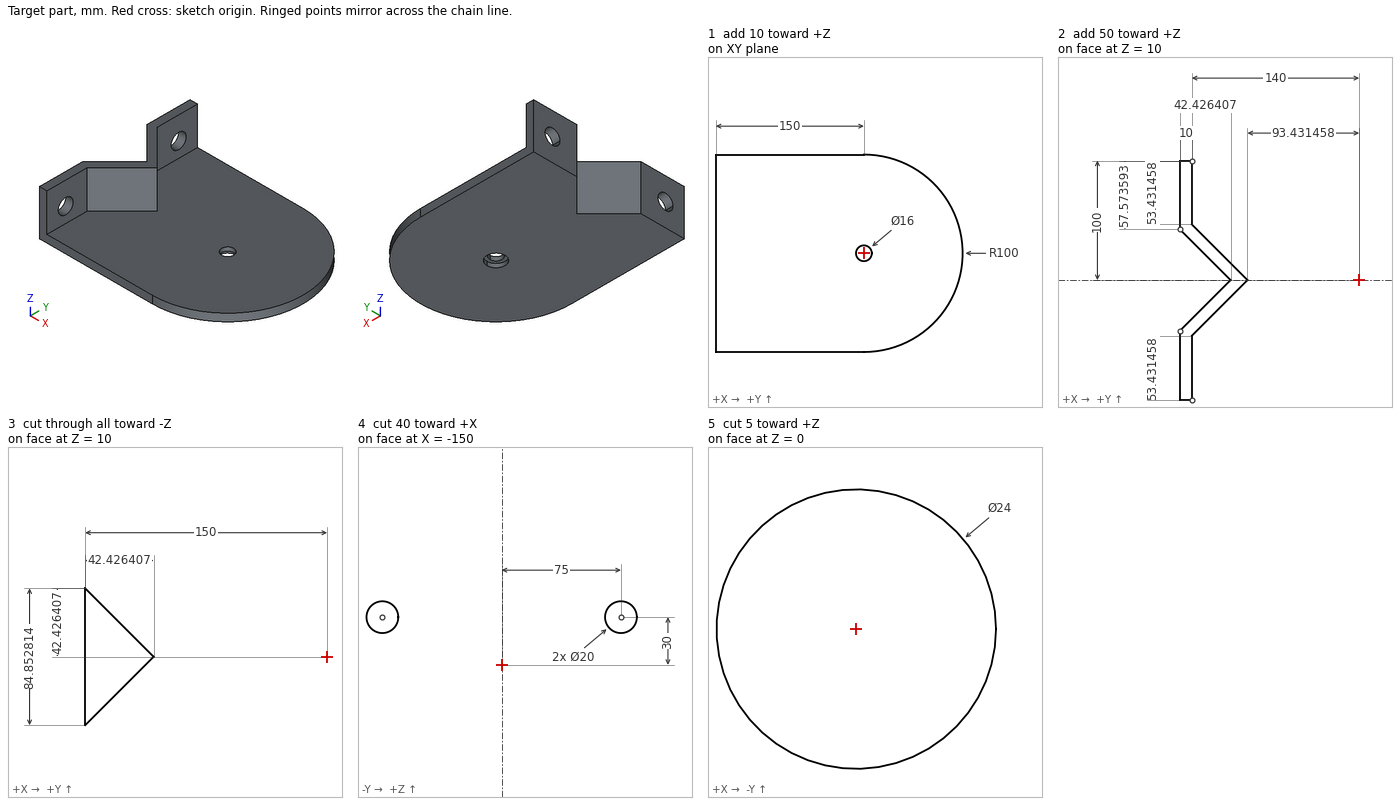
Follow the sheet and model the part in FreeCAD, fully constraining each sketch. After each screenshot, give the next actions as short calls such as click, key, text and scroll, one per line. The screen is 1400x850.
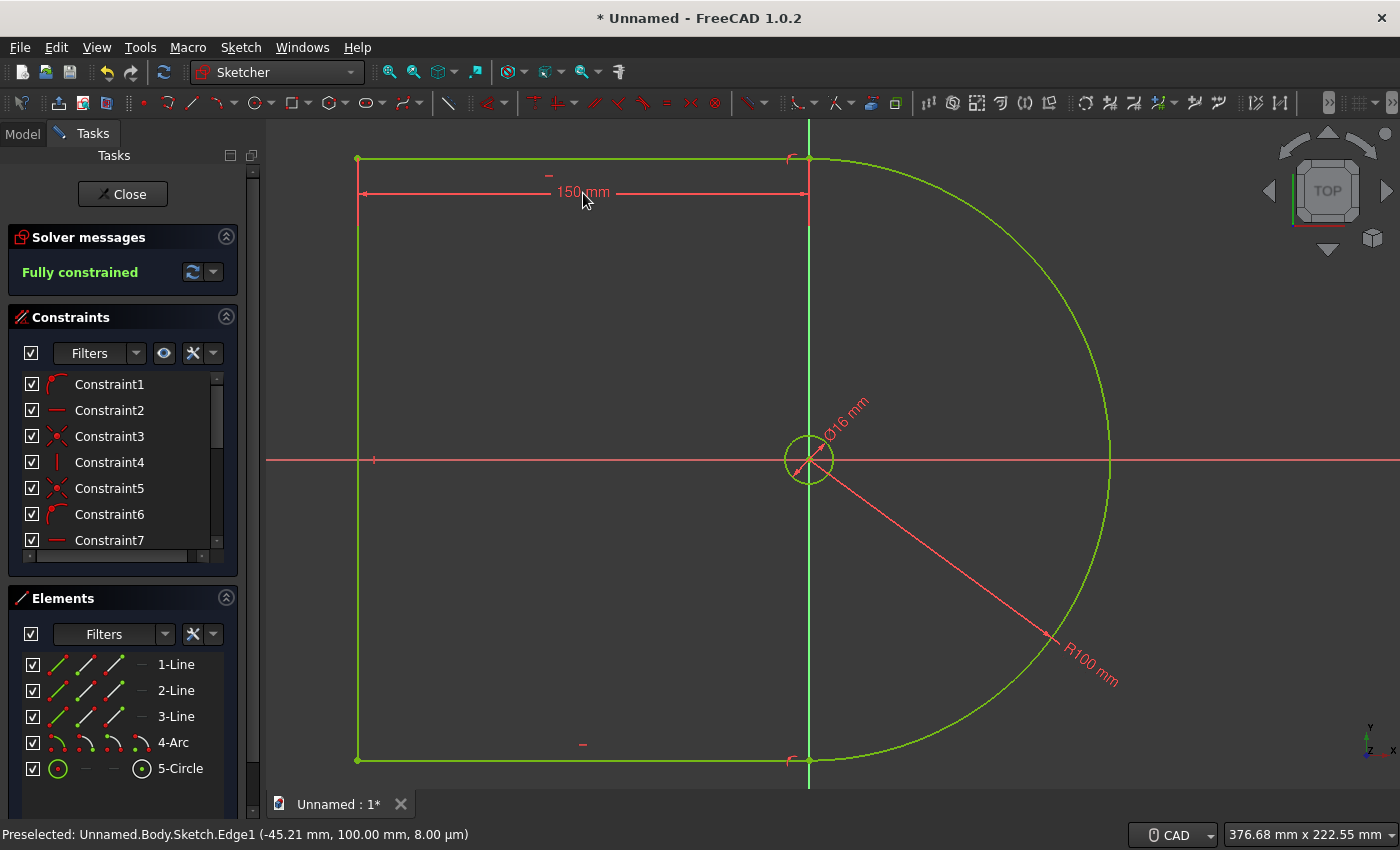
click(123, 194)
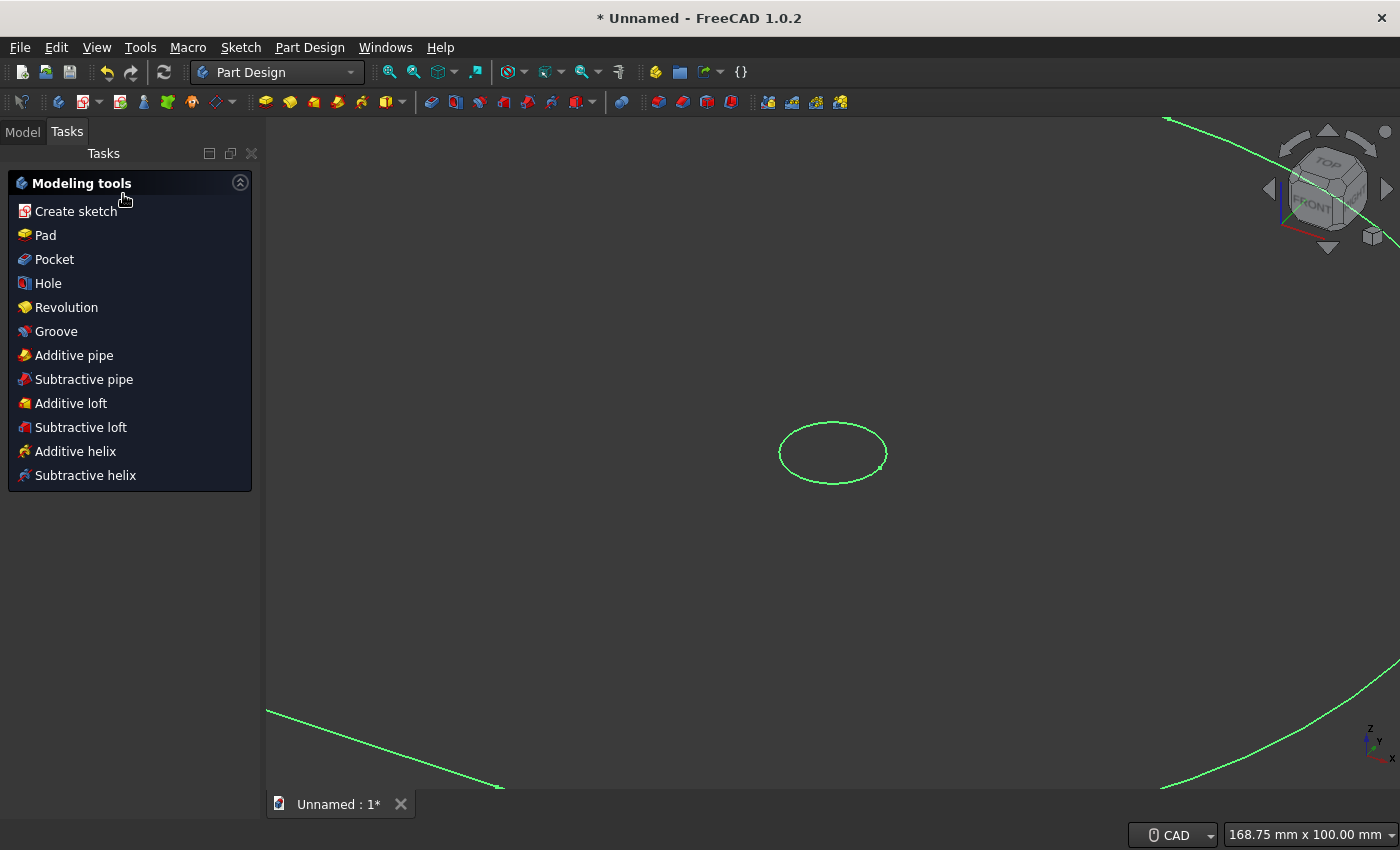
click(266, 102)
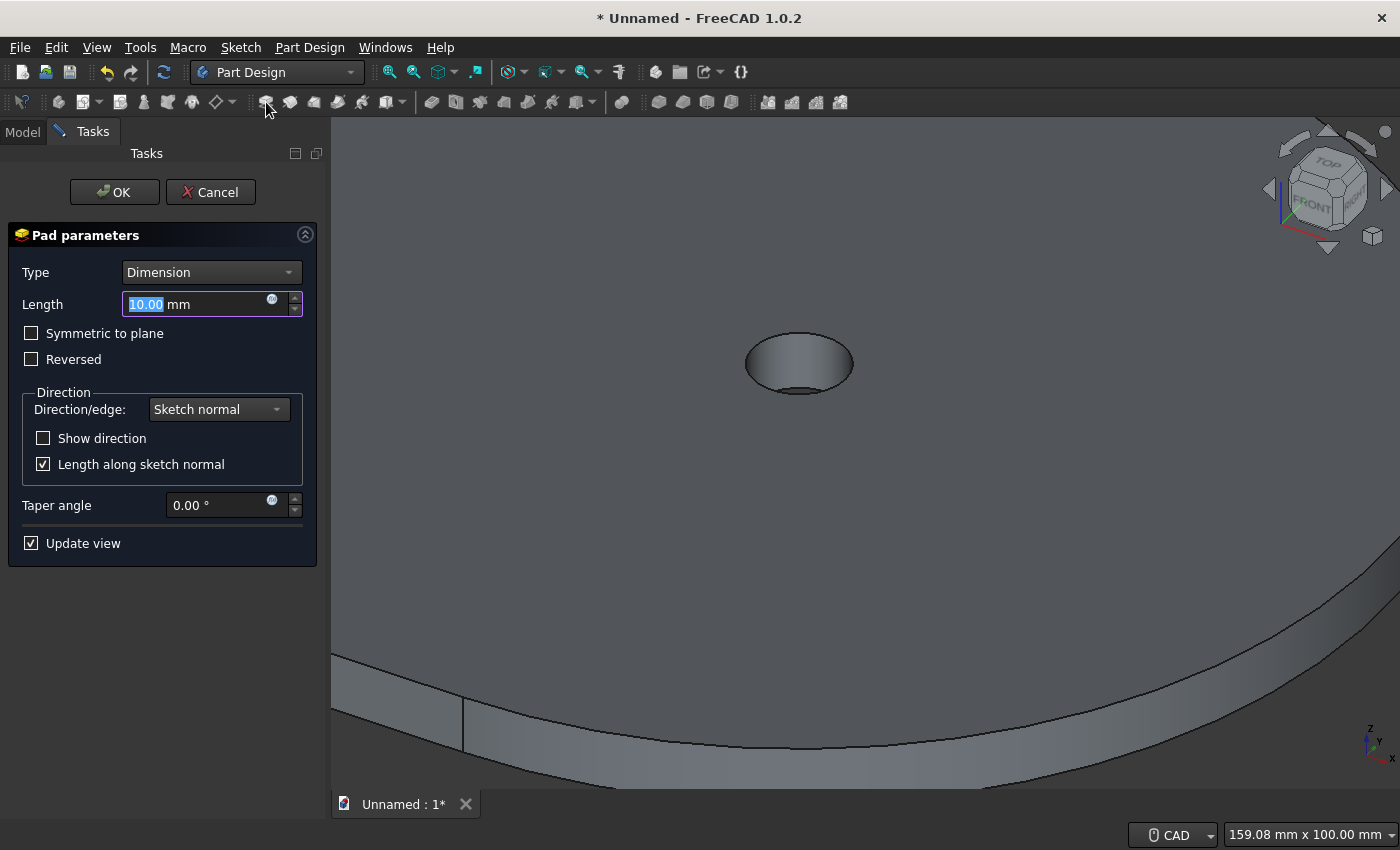
text(10)
key(Tab)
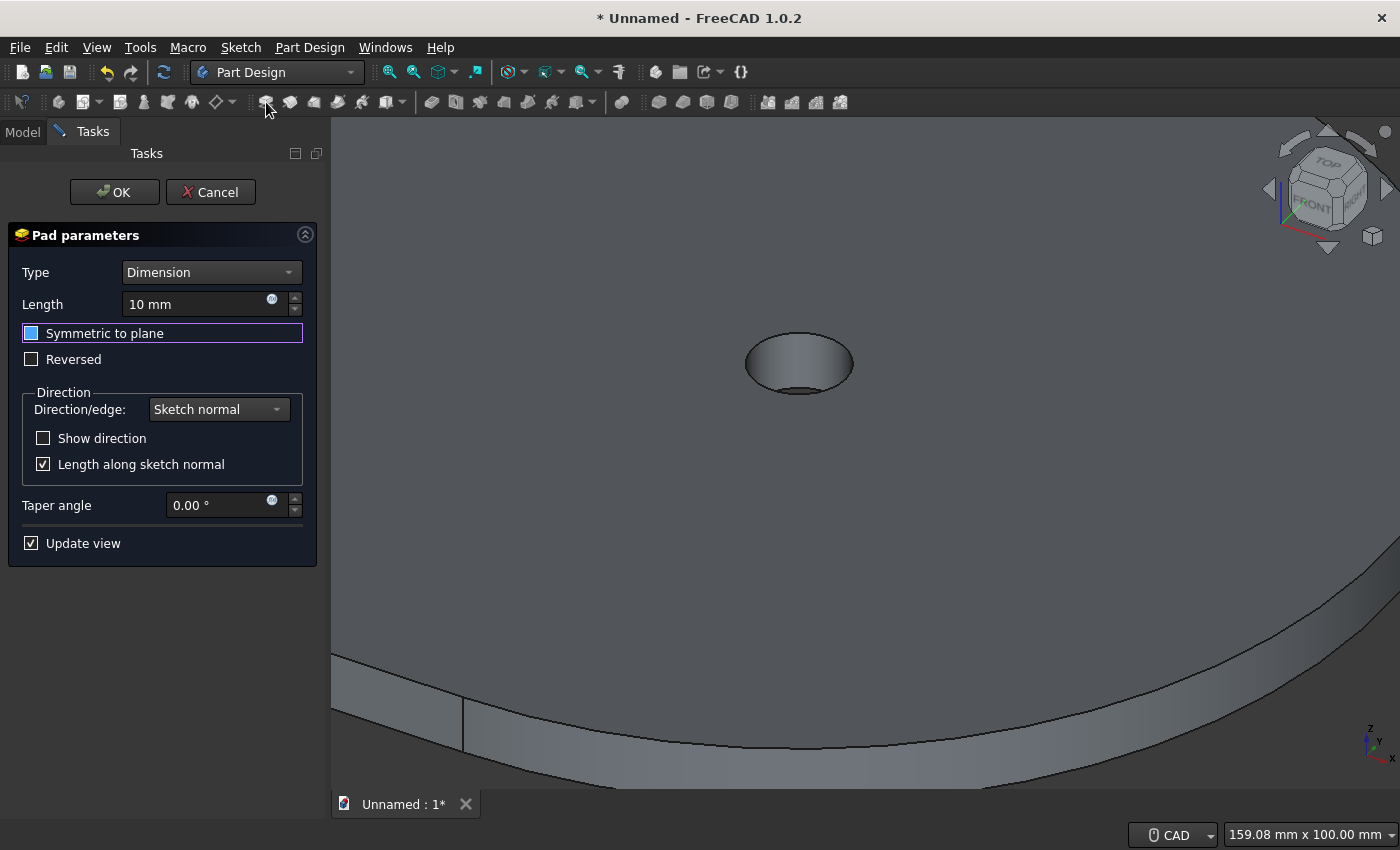
click(115, 192)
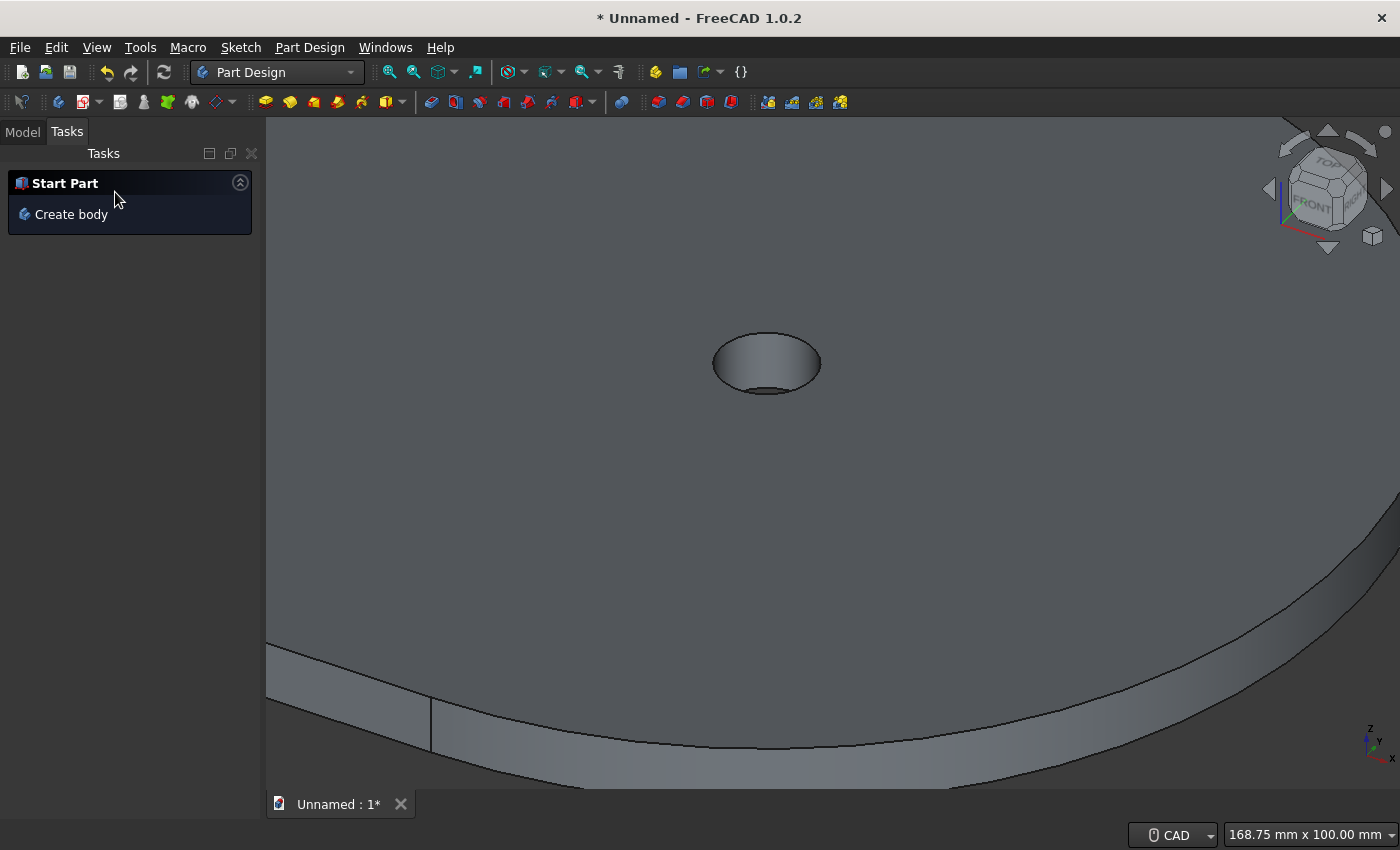
click(390, 72)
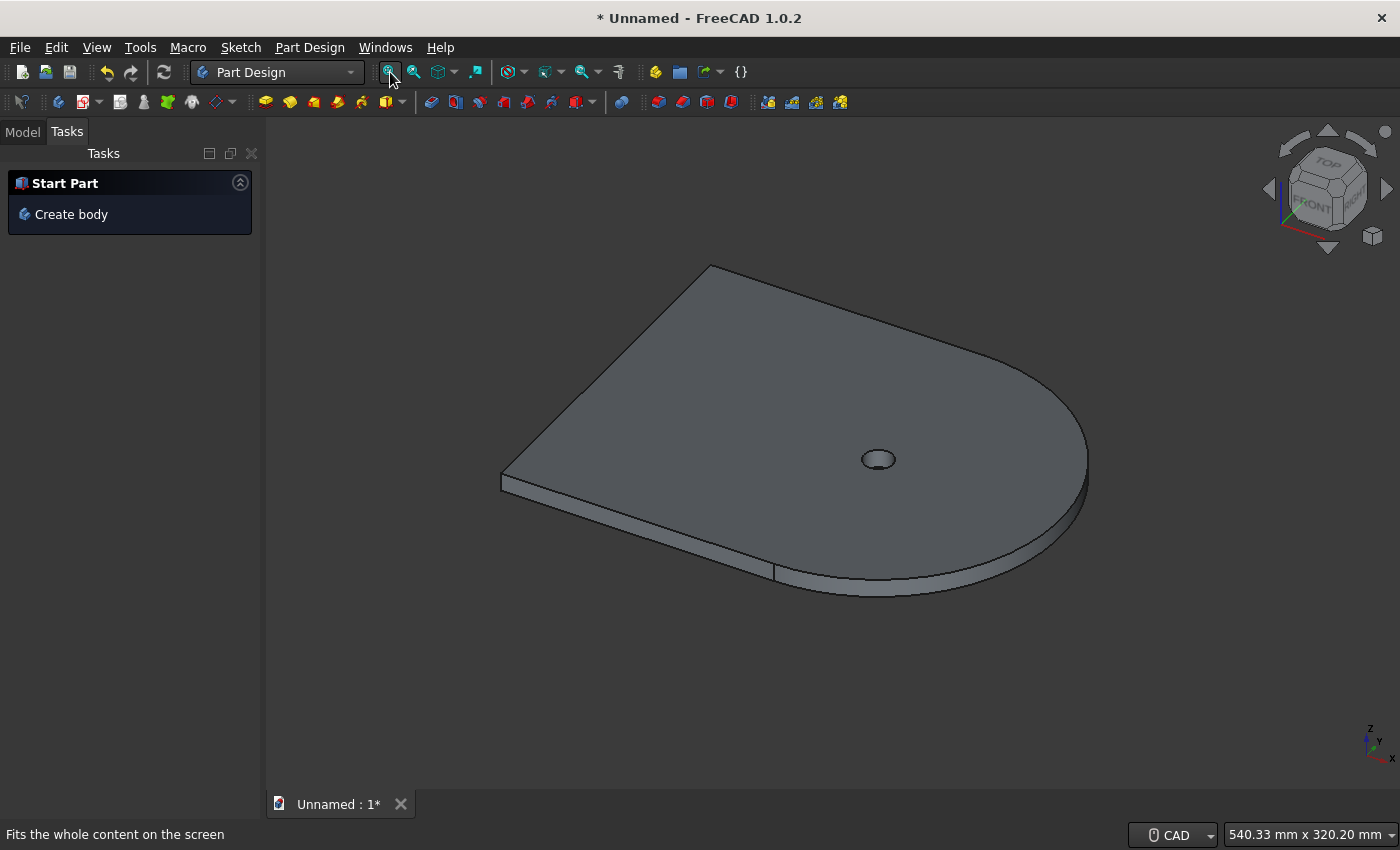
click(798, 392)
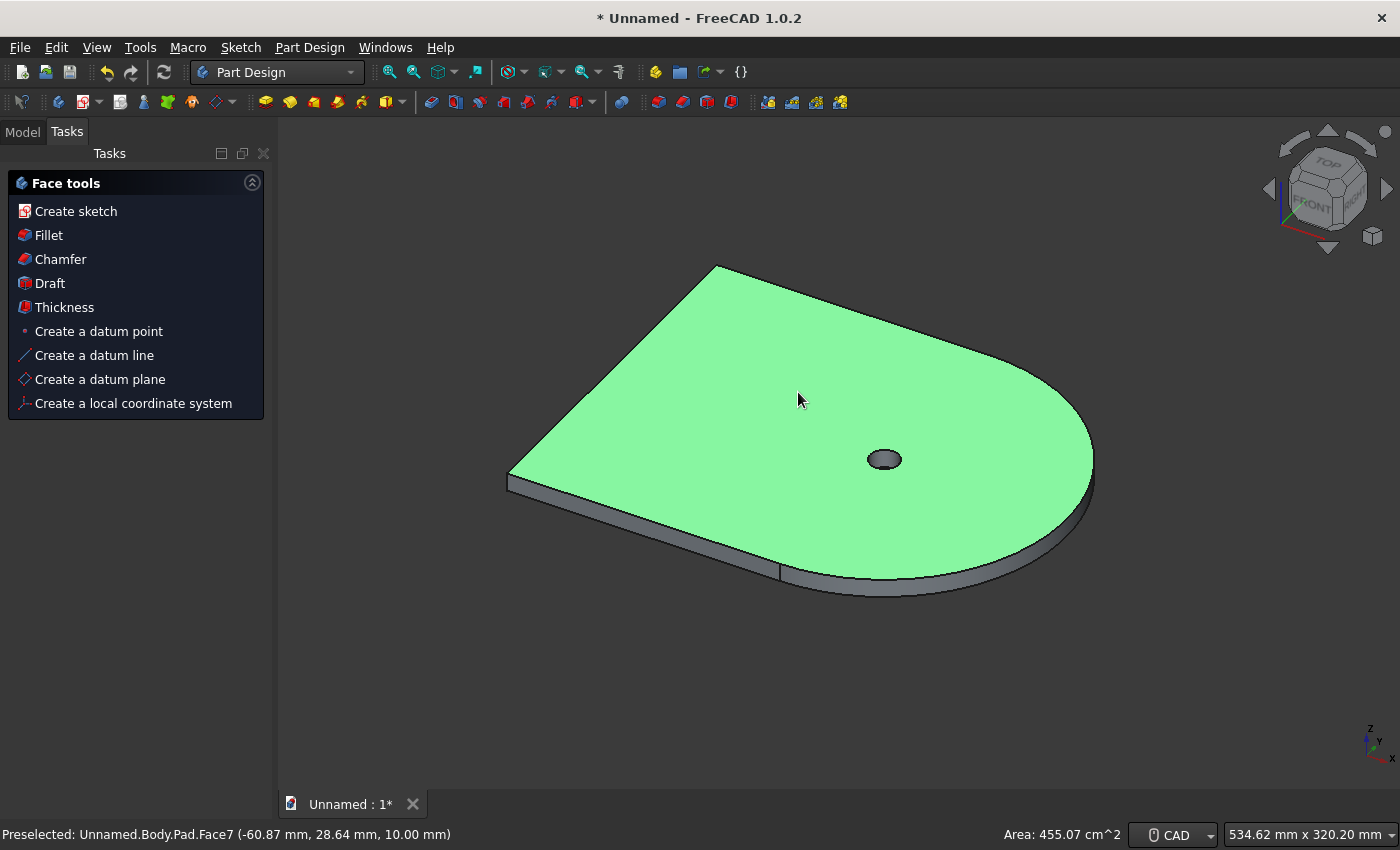
click(84, 102)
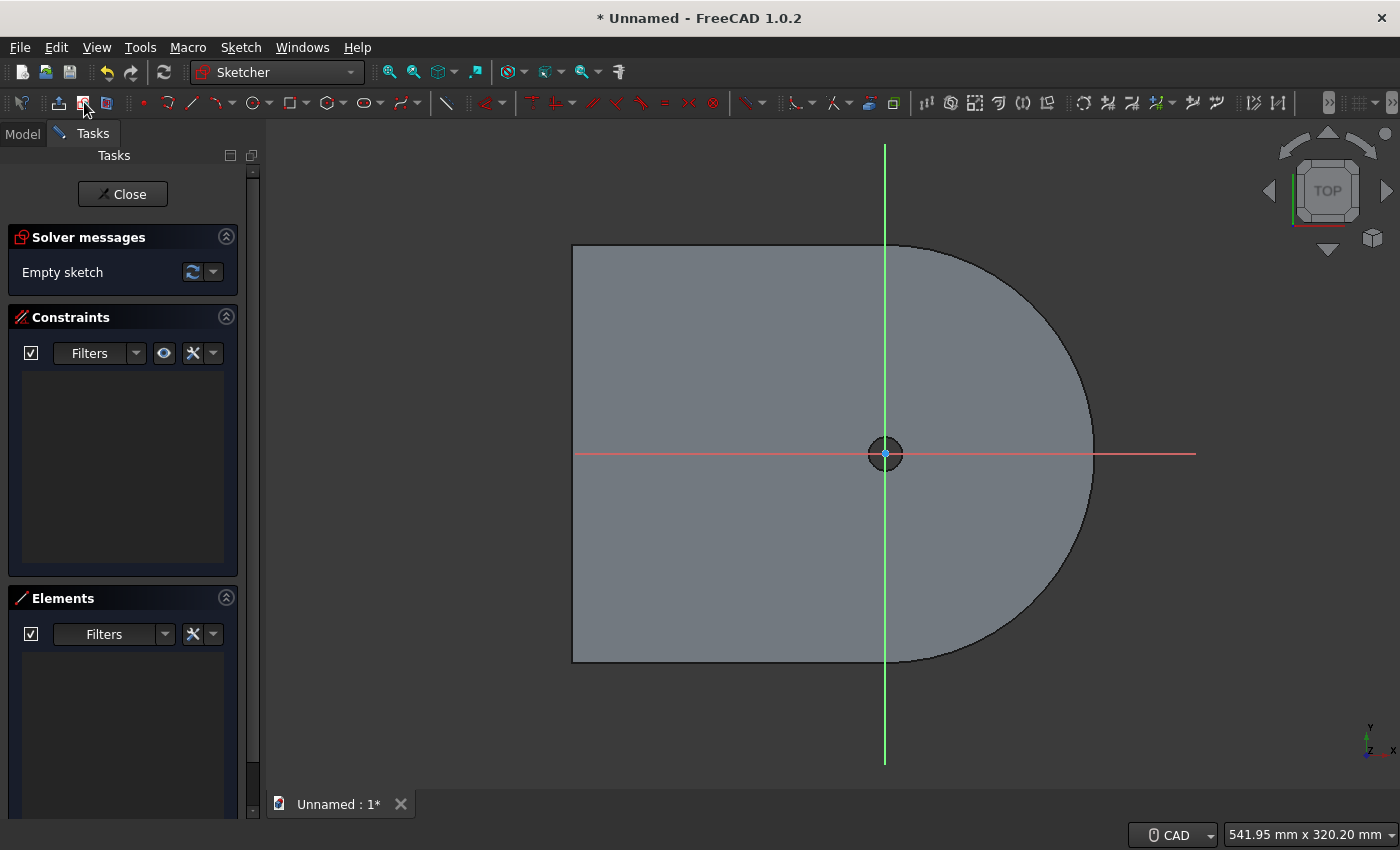
key(g)
key(m)